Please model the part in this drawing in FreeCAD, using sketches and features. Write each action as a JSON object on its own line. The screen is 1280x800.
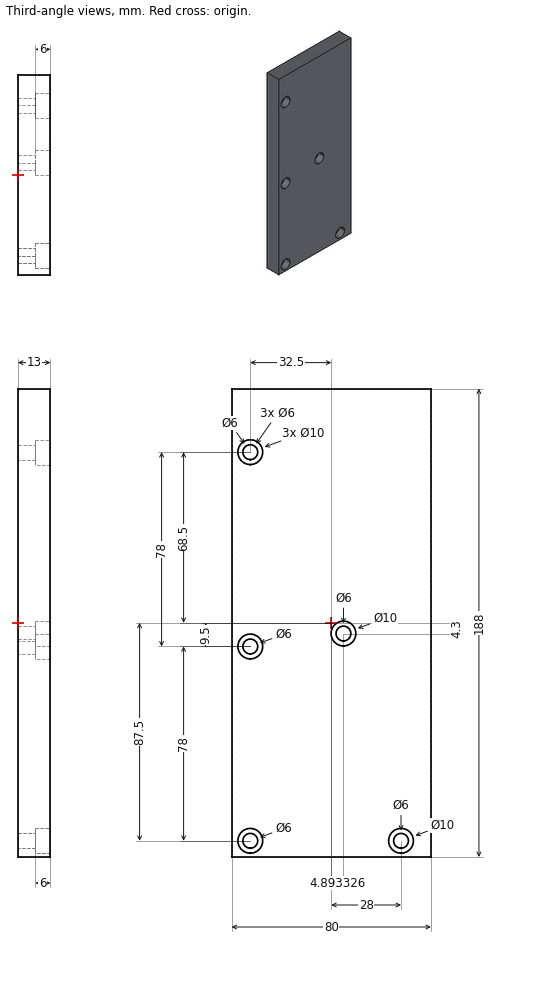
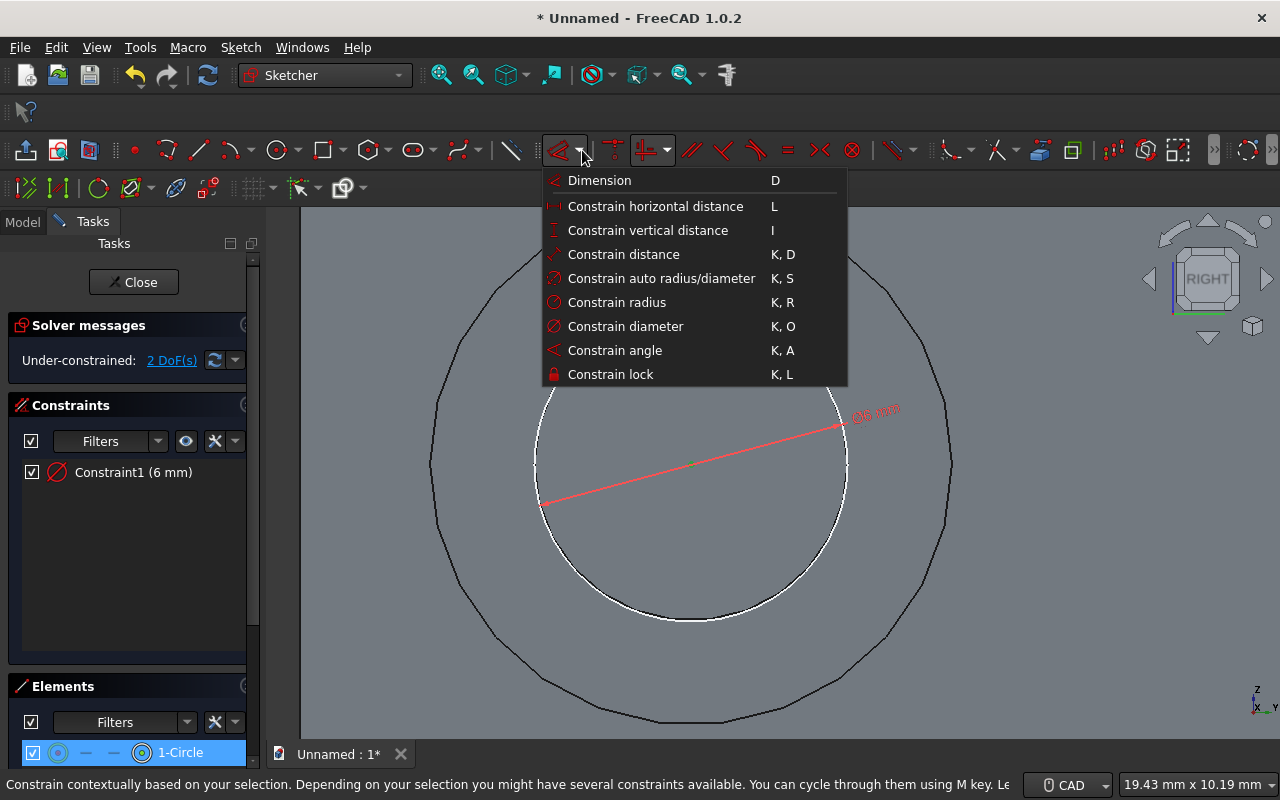
{"action": "left_click", "coordinate": [695, 206]}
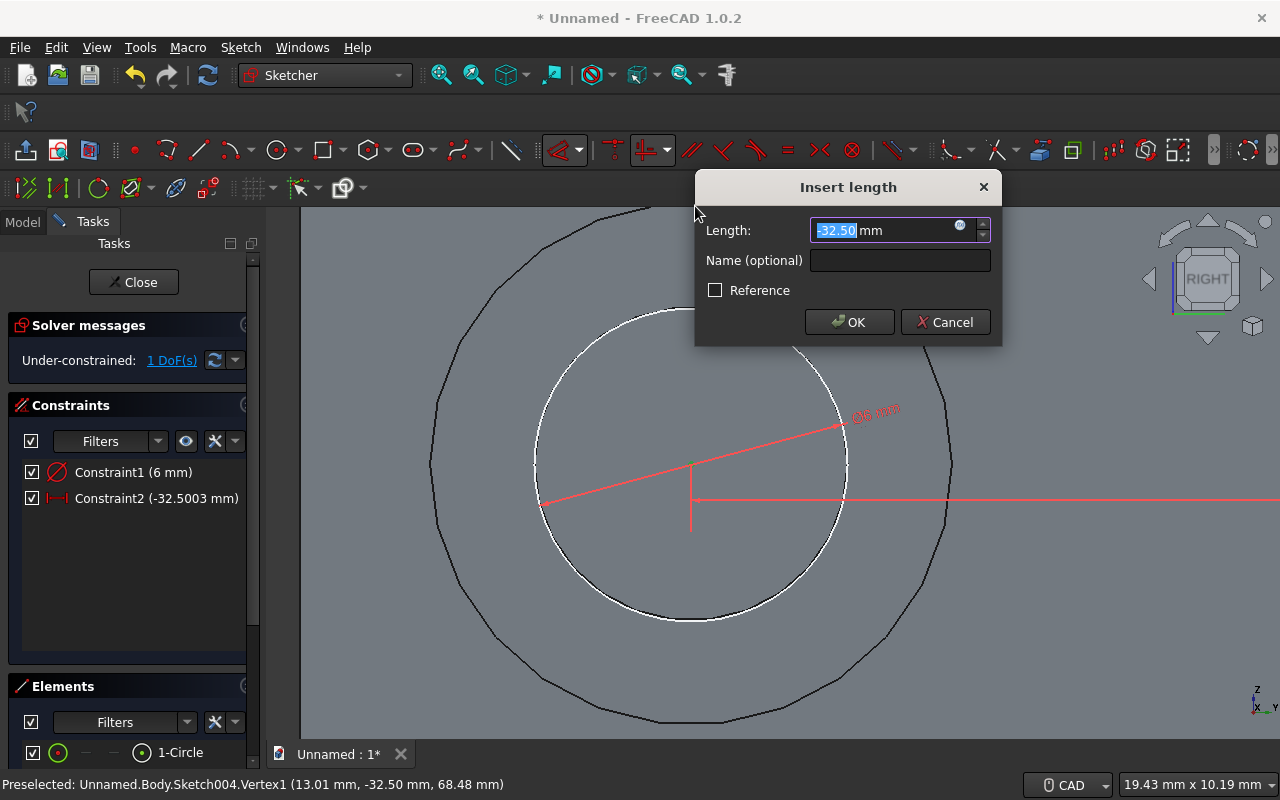
{"action": "type", "text": "-32.5"}
{"action": "key", "text": "Return"}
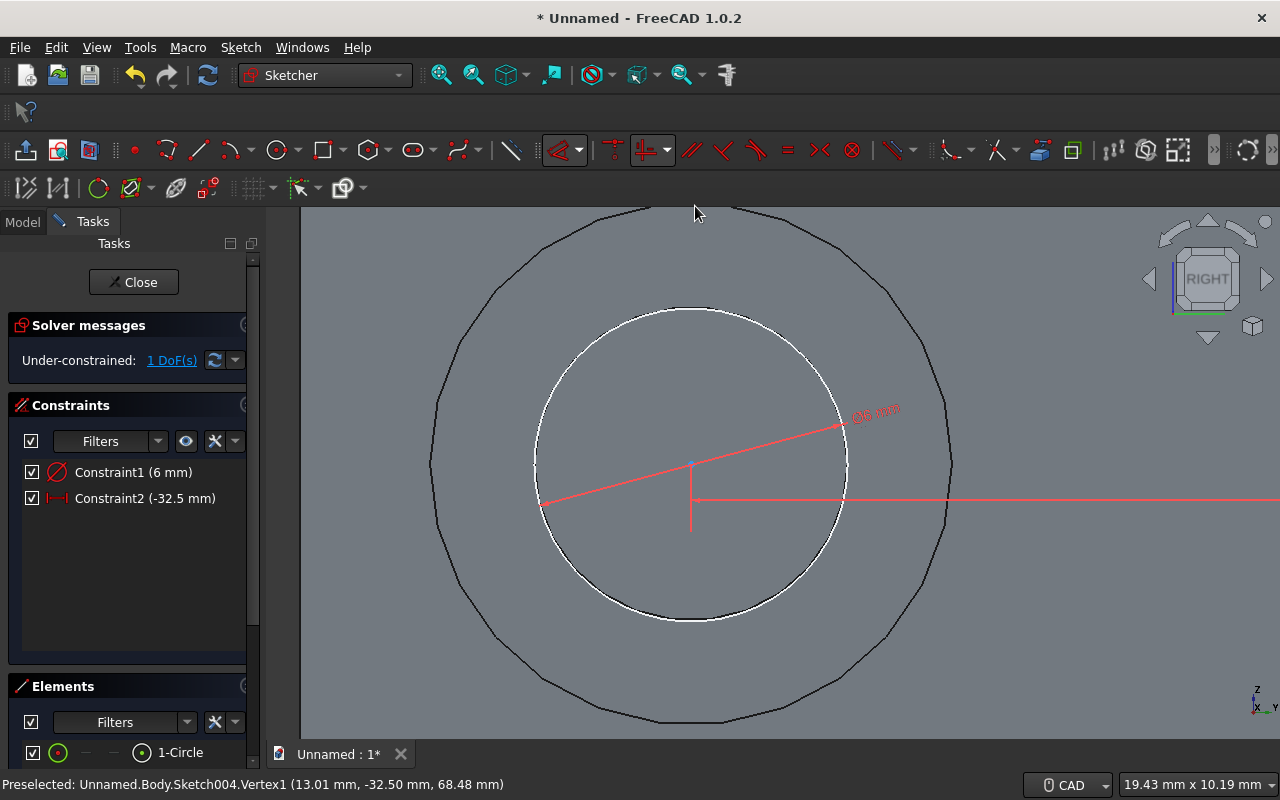
{"action": "left_click", "coordinate": [691, 465]}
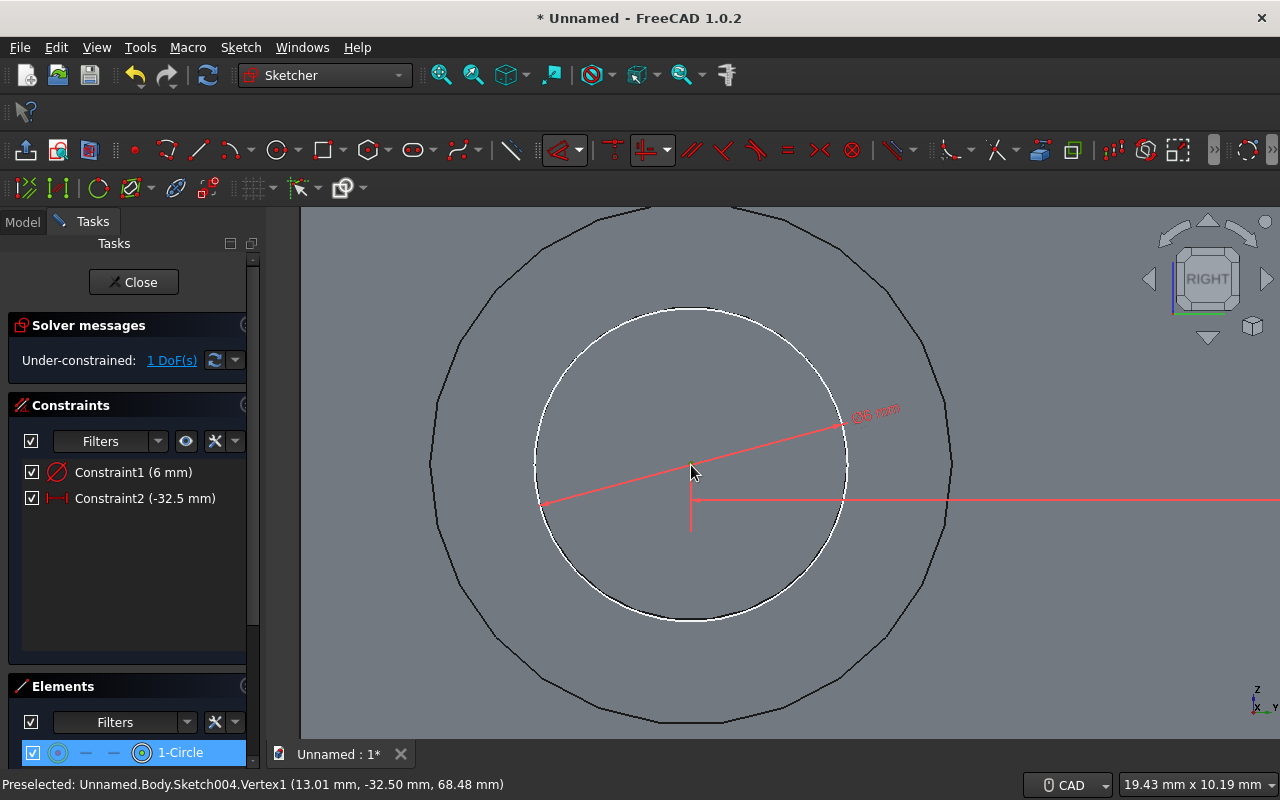
{"action": "key", "text": "i"}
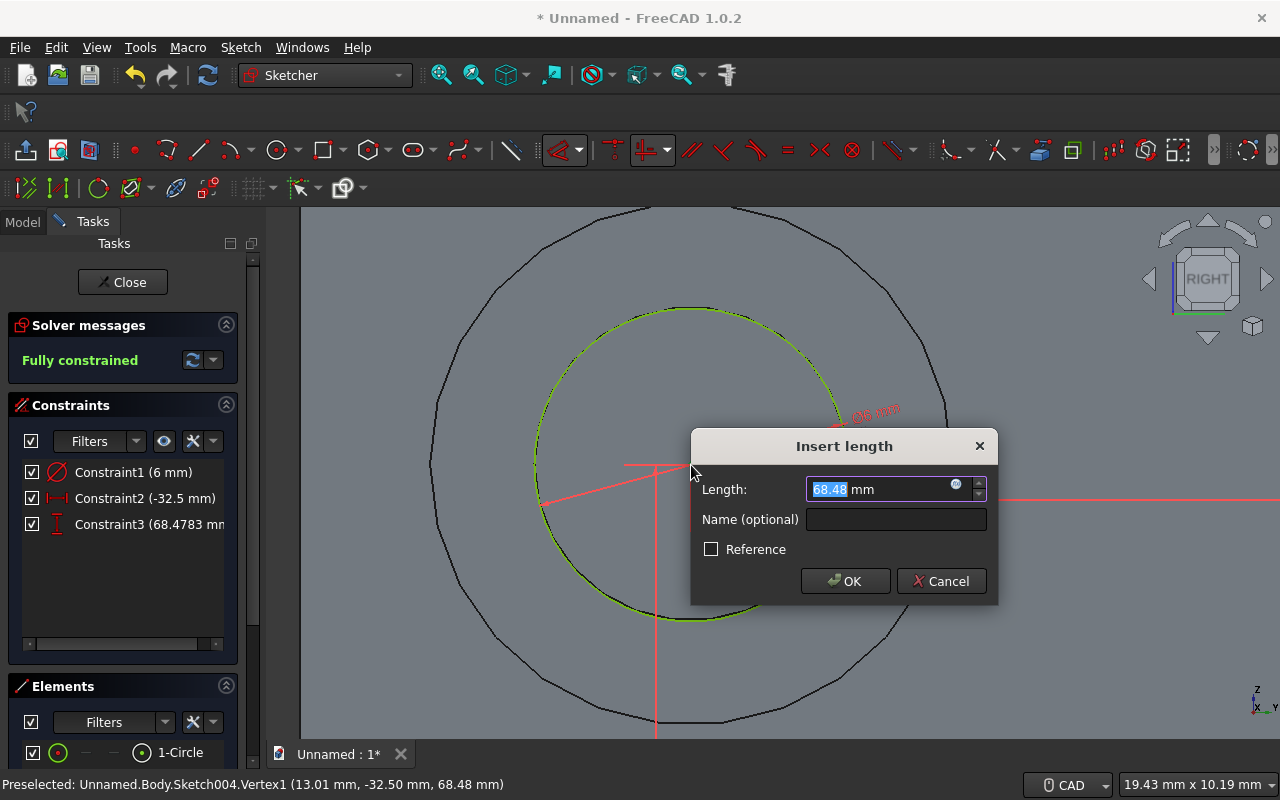
{"action": "type", "text": "68.5"}
{"action": "key", "text": "Return"}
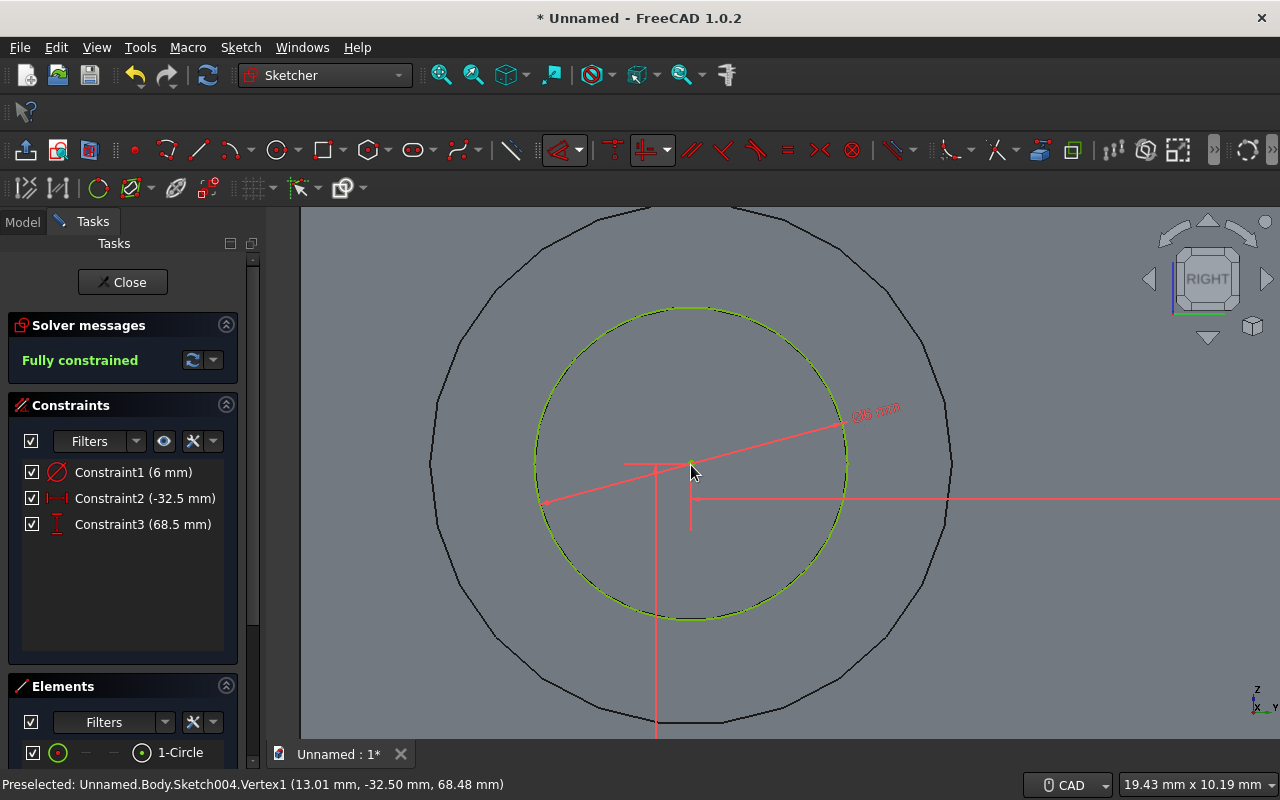
{"action": "left_click", "coordinate": [123, 282]}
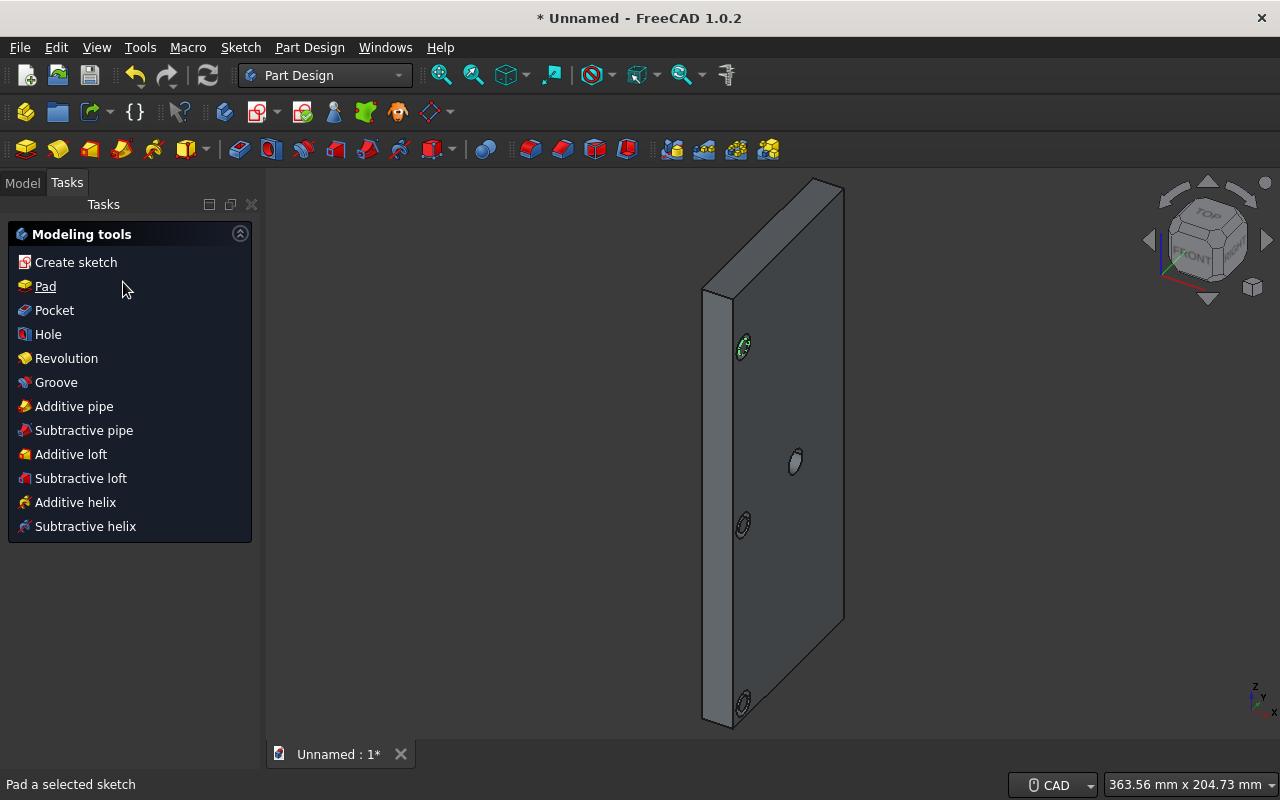
{"action": "left_click", "coordinate": [240, 150]}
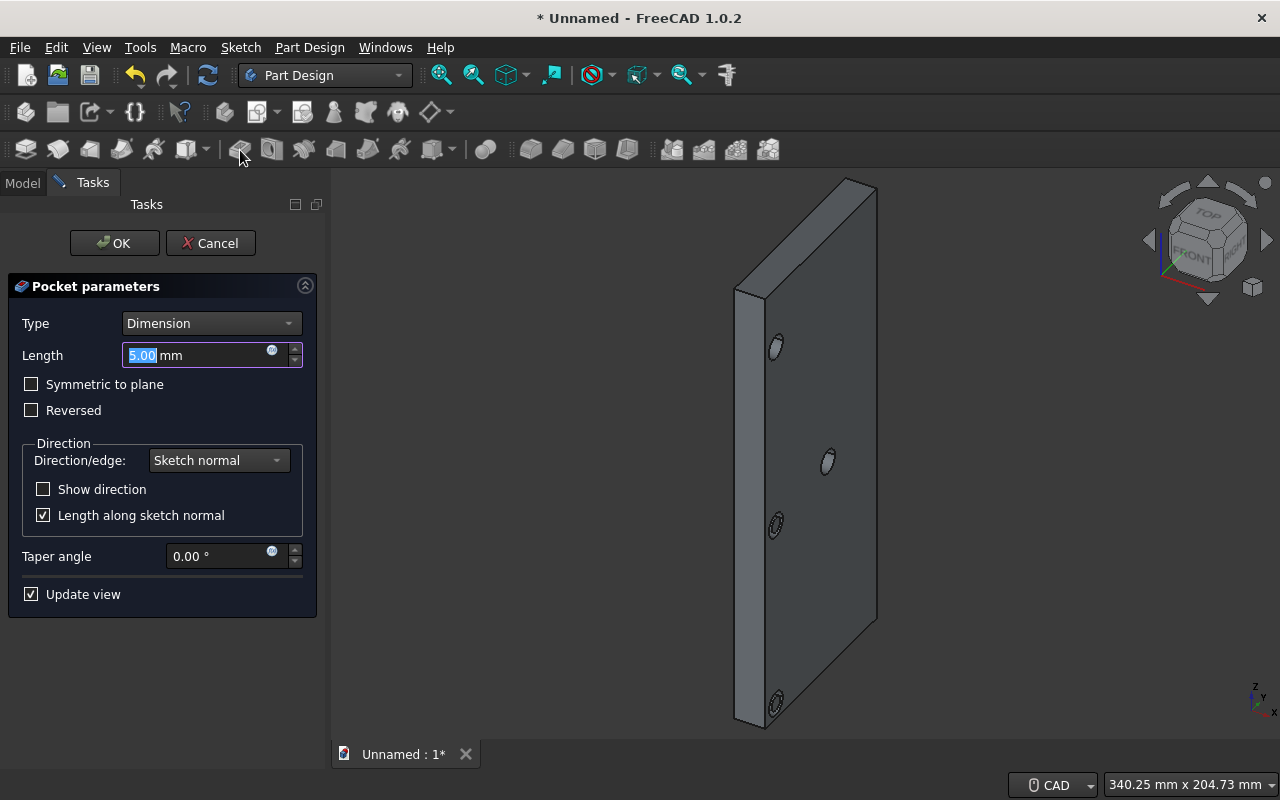
{"action": "left_click", "coordinate": [212, 324]}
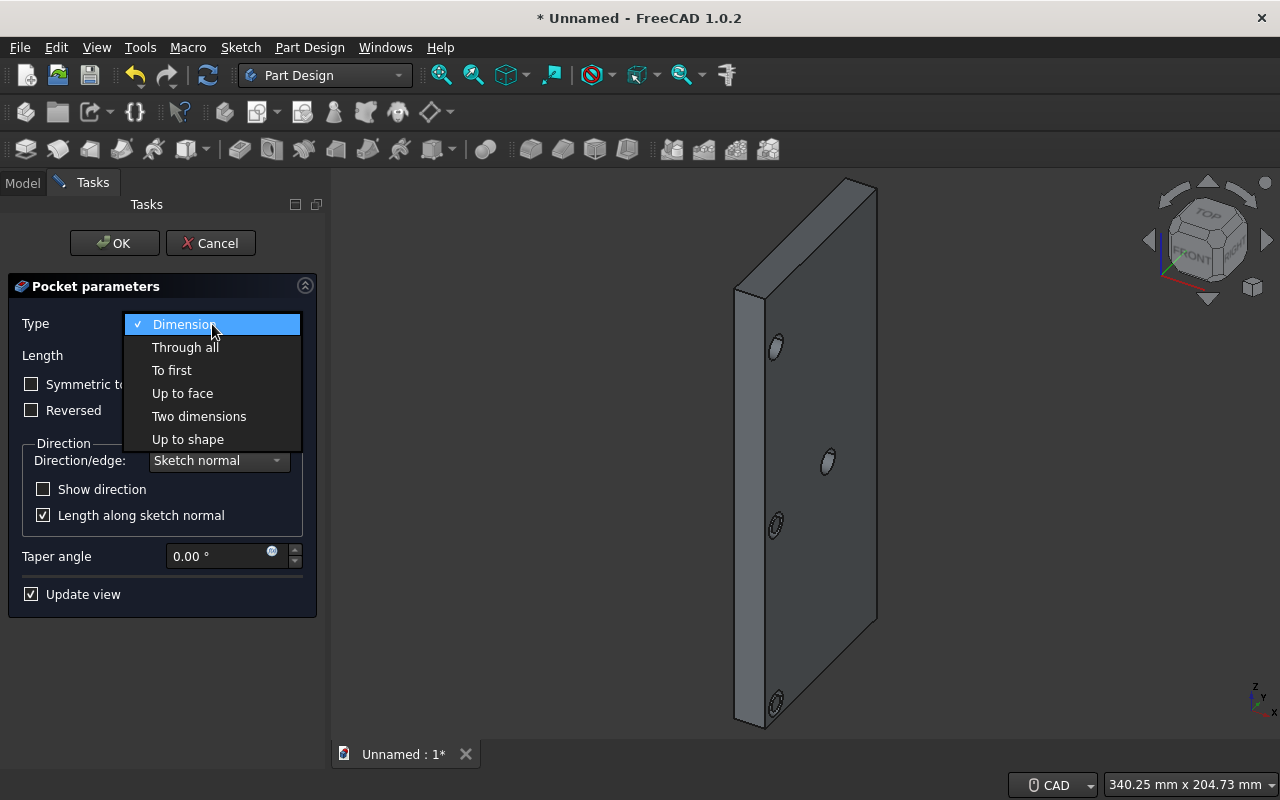
{"action": "left_click", "coordinate": [212, 370]}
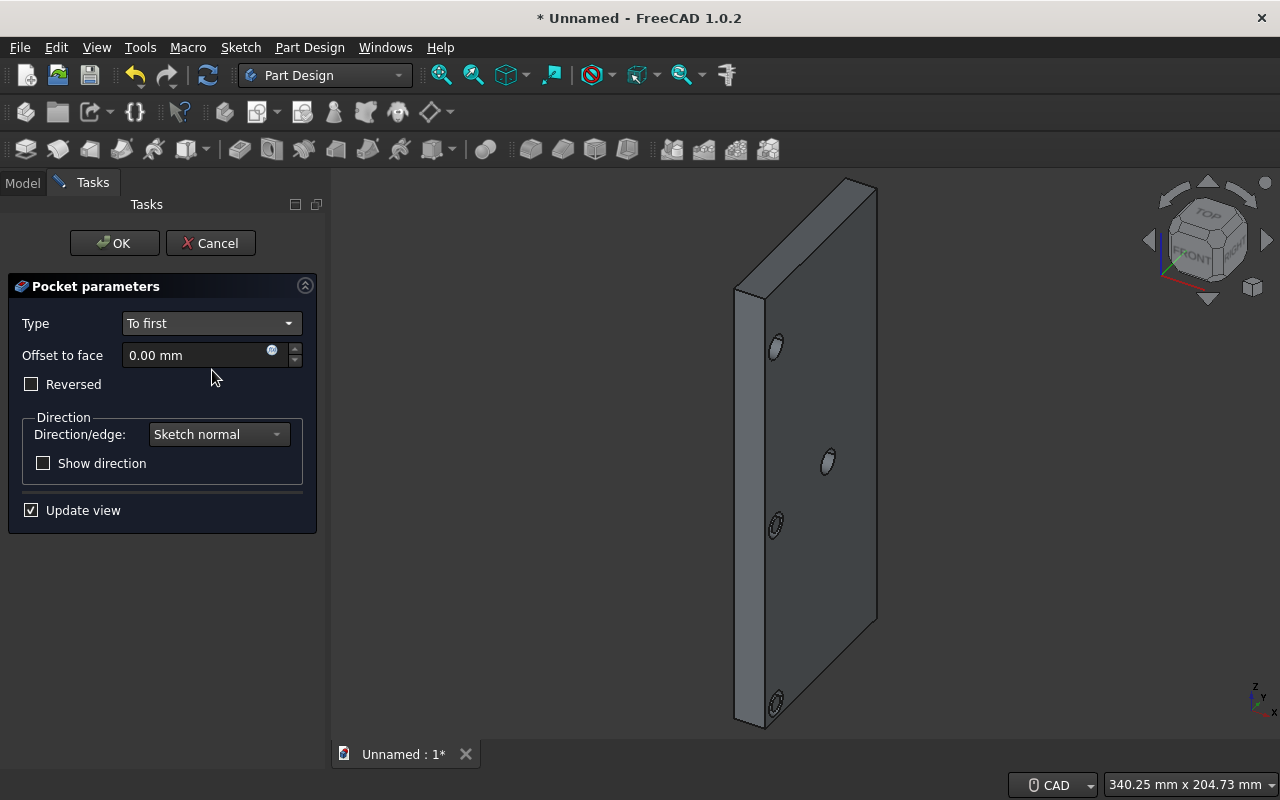
{"action": "left_click", "coordinate": [115, 243]}